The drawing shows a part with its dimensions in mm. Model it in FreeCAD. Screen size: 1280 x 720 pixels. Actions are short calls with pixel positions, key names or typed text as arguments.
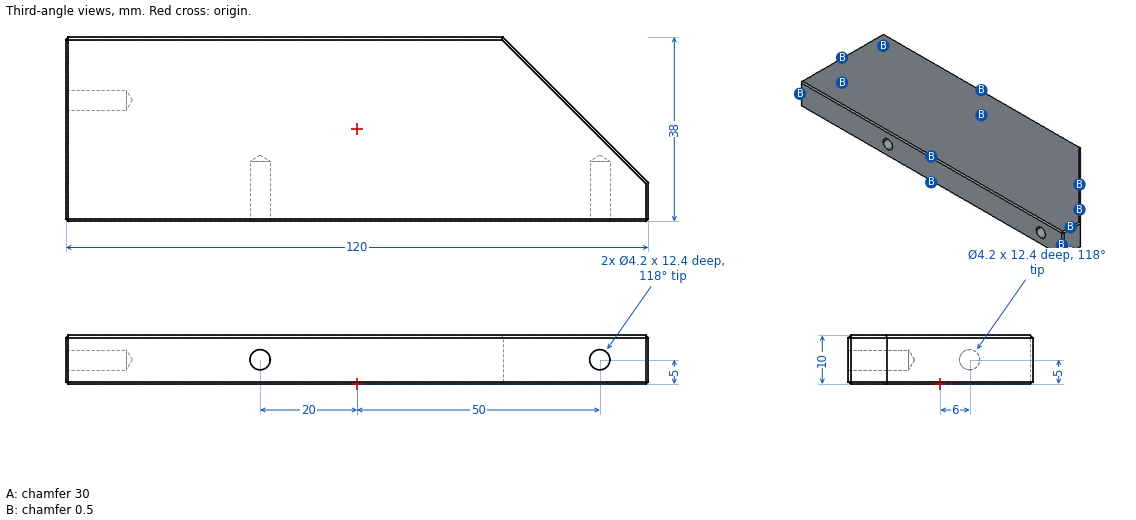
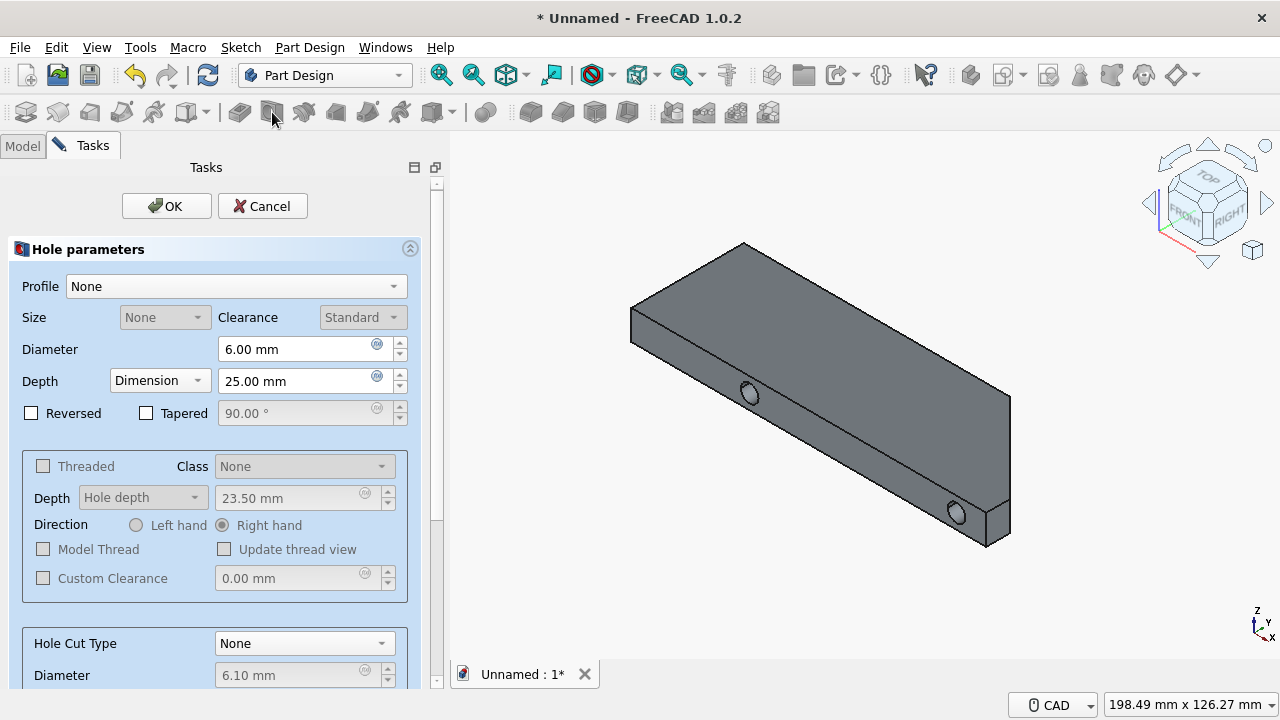
triple_click(305, 349)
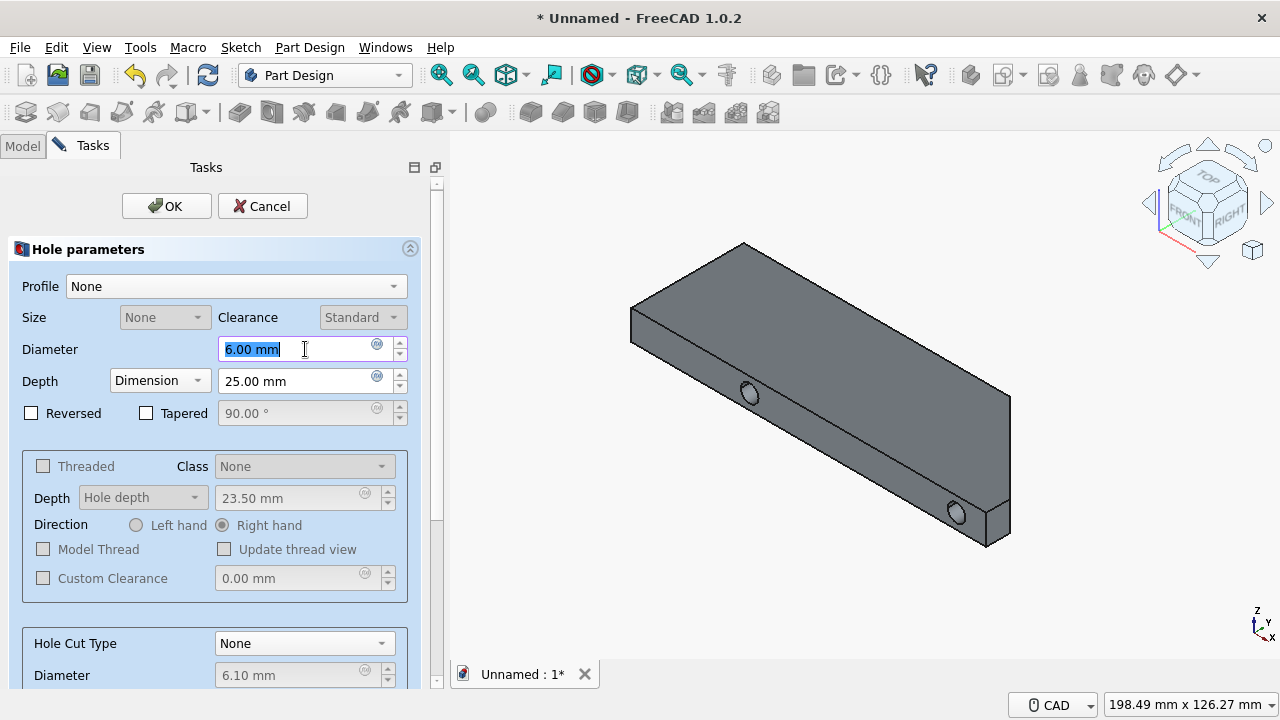
text(4.2)
key(Tab)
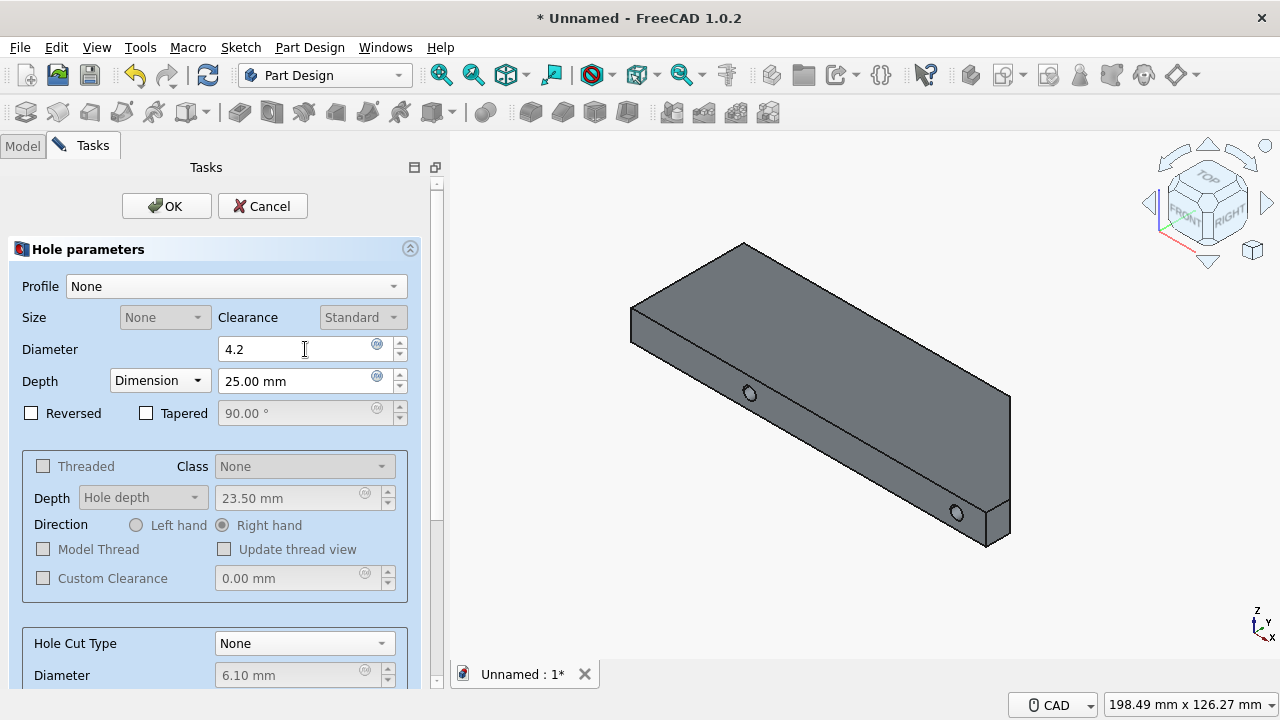
triple_click(305, 381)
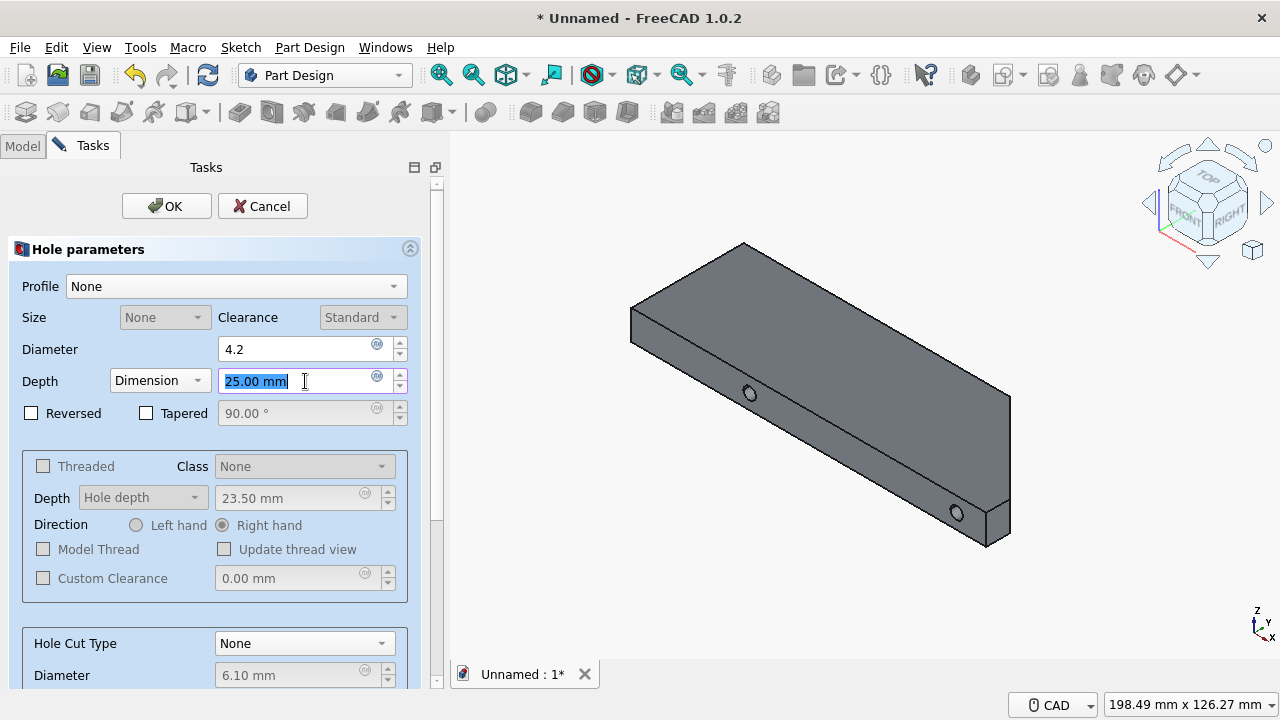
text(12.4)
key(Tab)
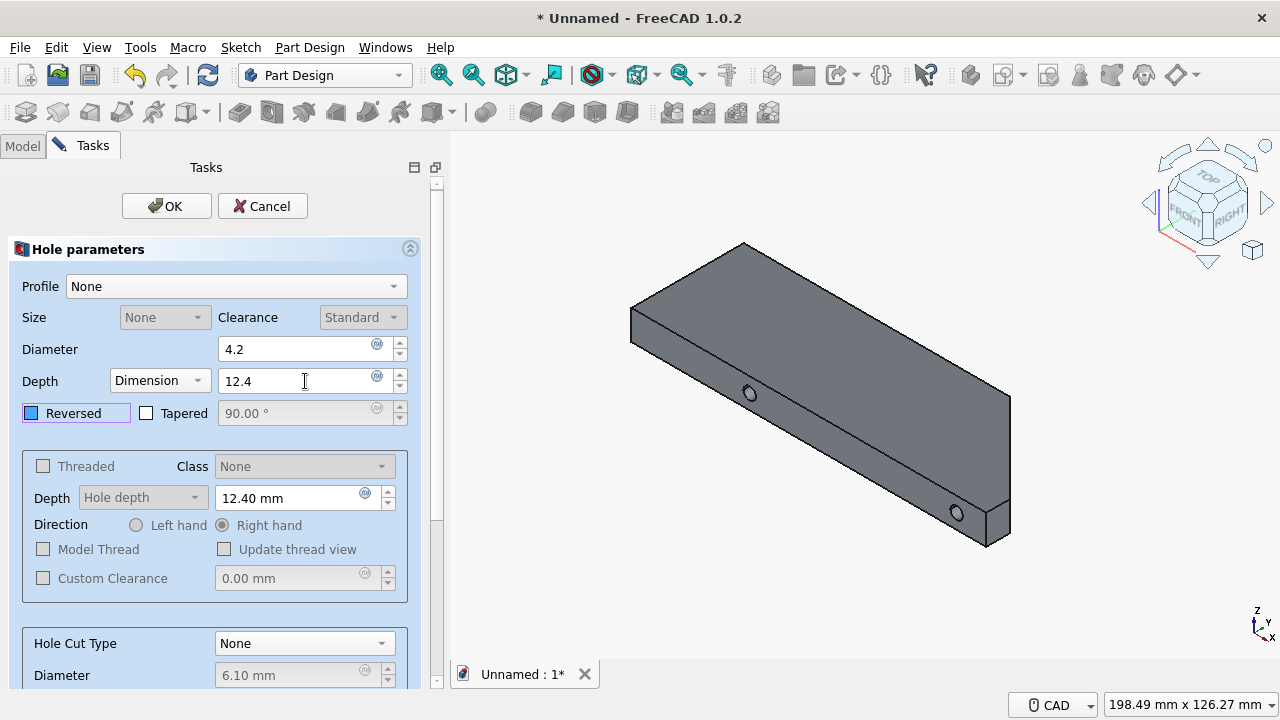
click(167, 206)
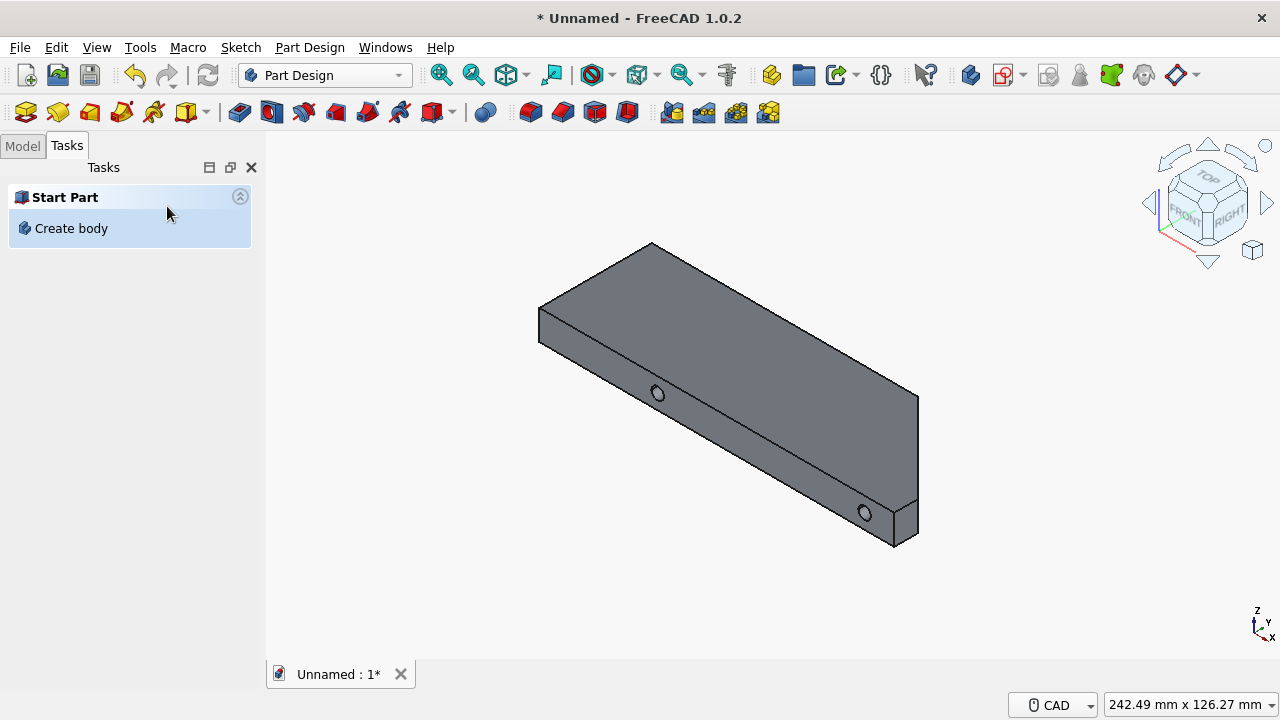
click(824, 406)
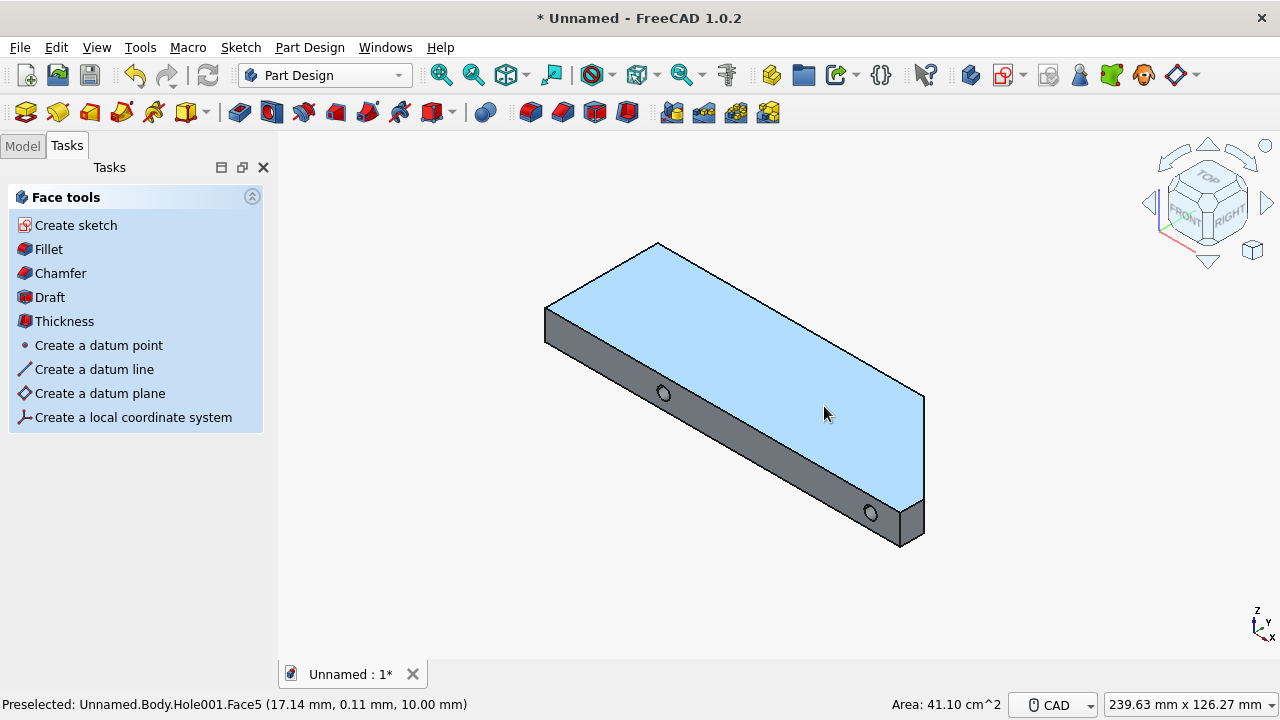
click(900, 529, ctrl)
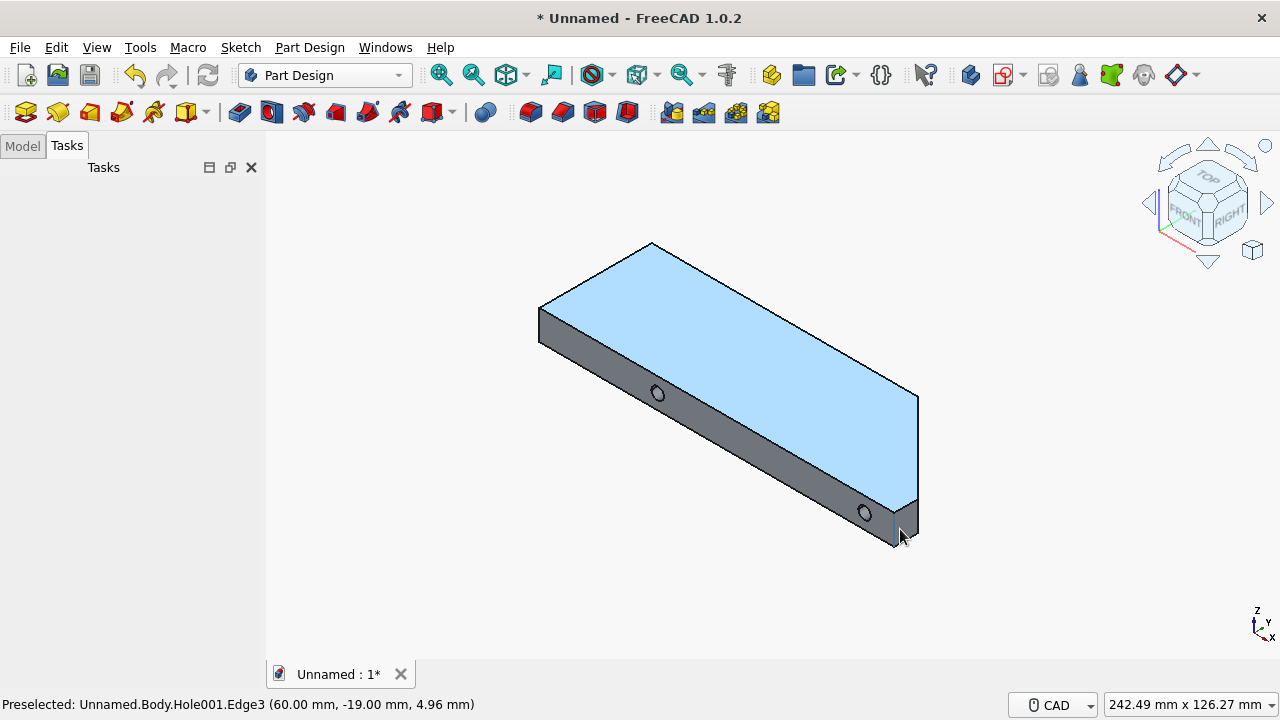
key(2)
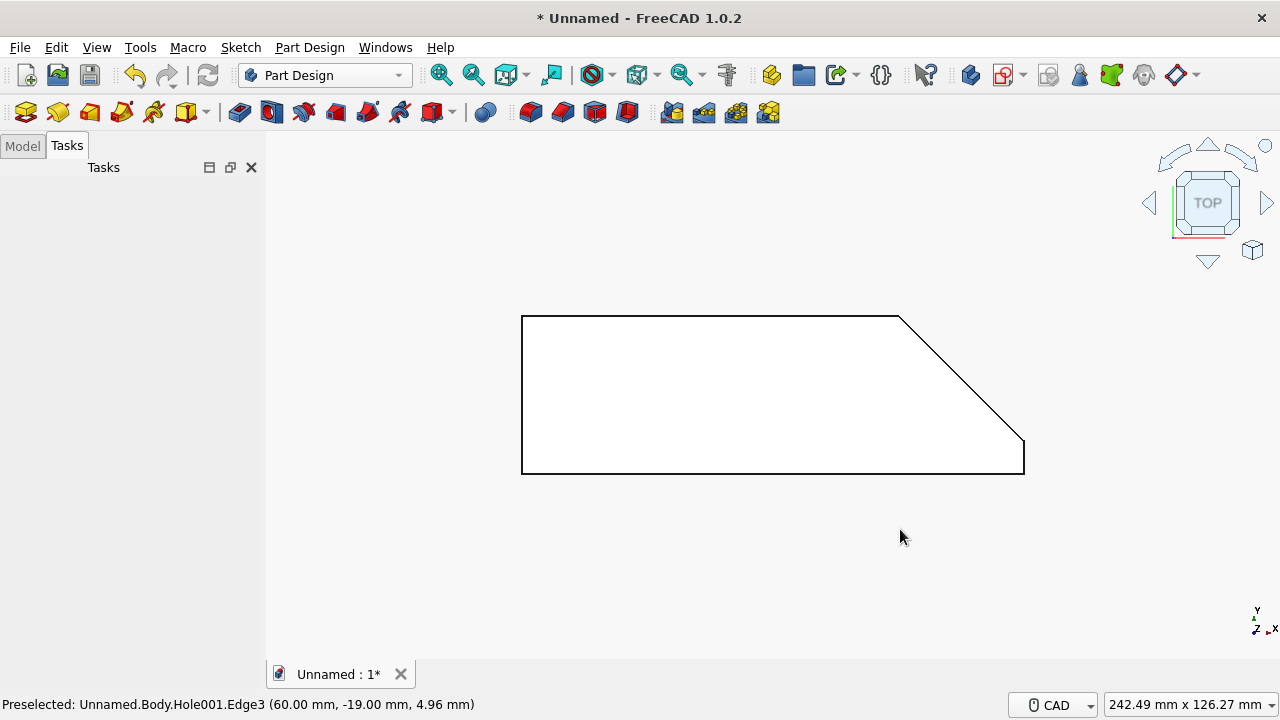
key(0)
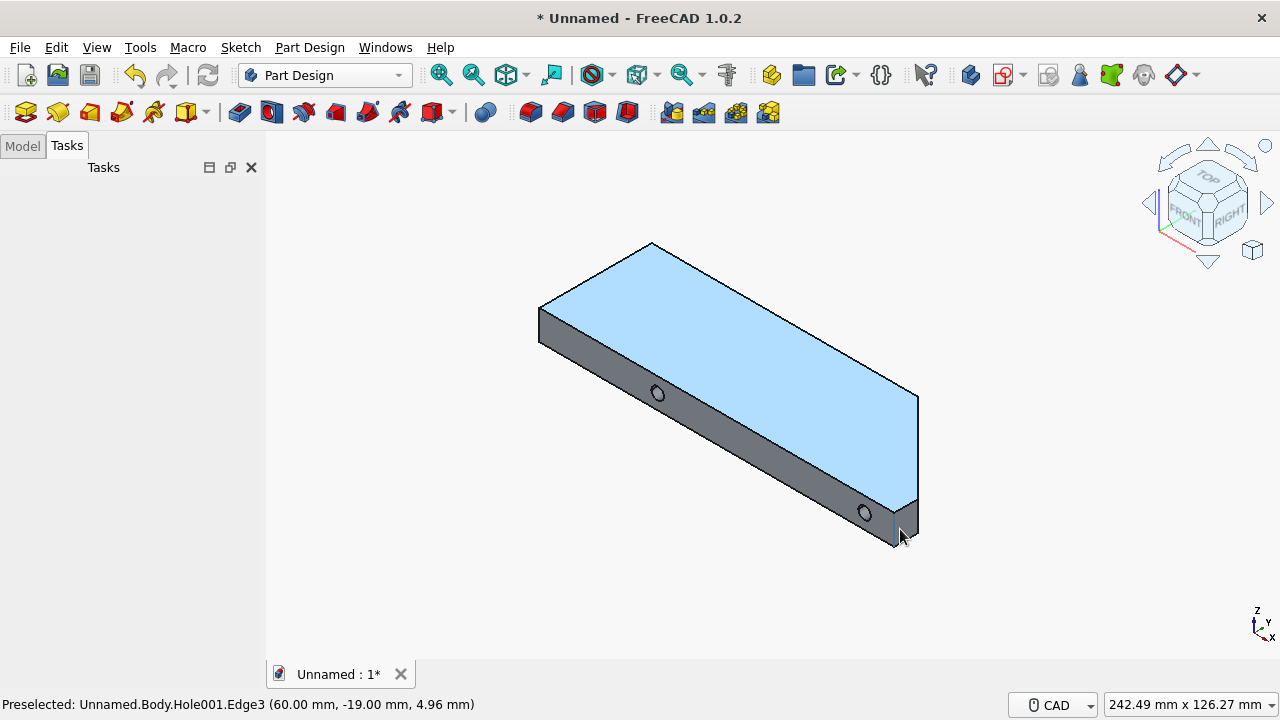
key(1)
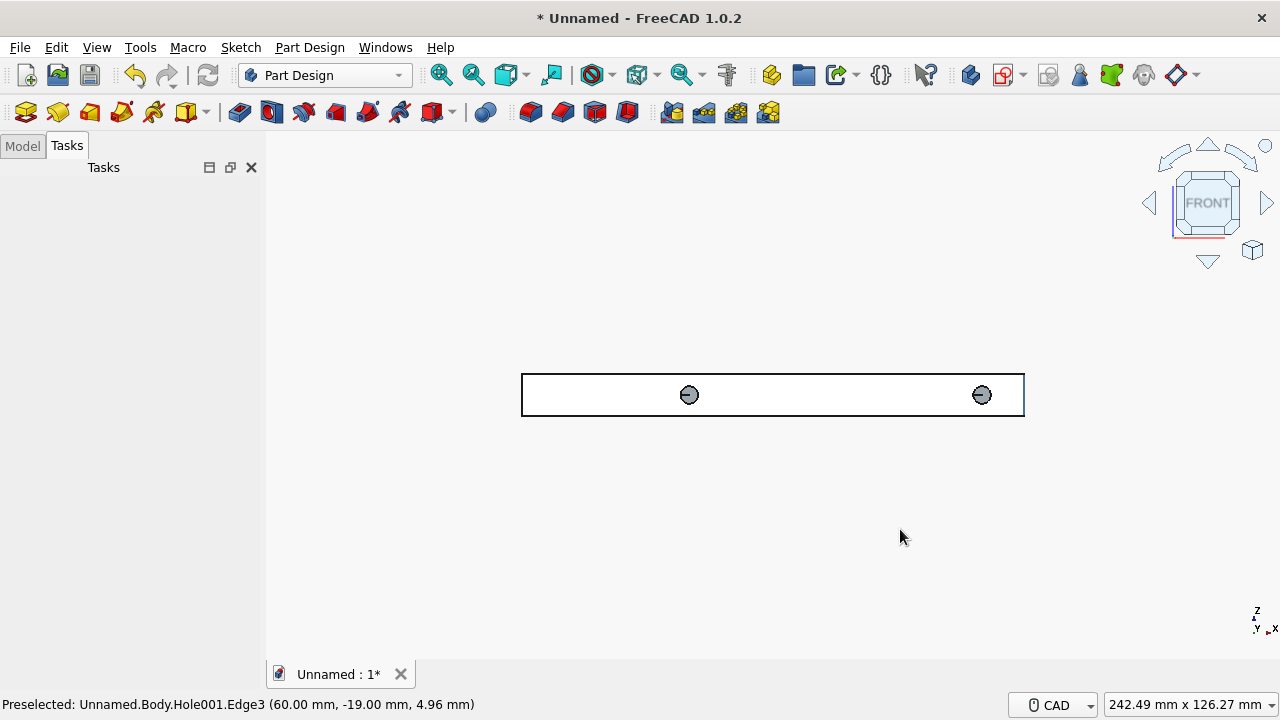
click(522, 394, ctrl)